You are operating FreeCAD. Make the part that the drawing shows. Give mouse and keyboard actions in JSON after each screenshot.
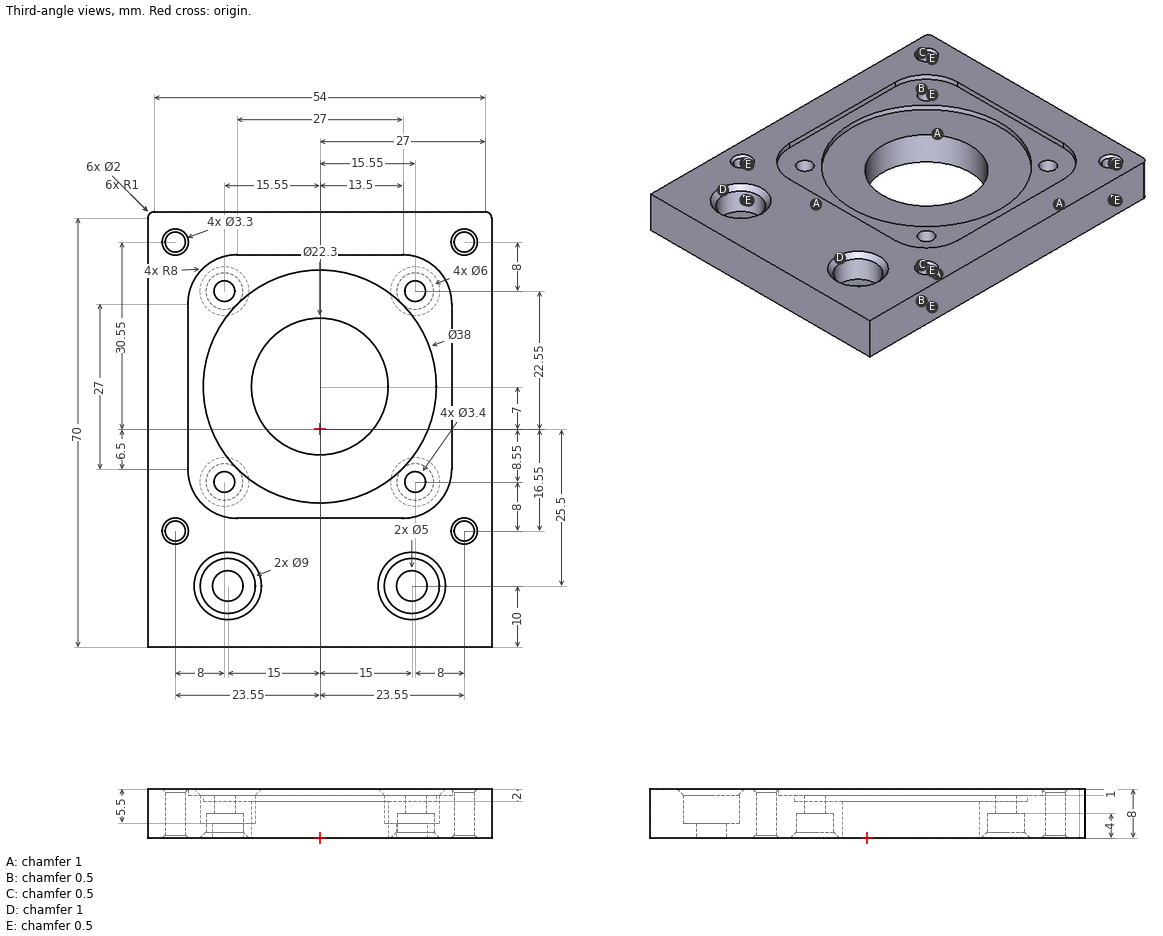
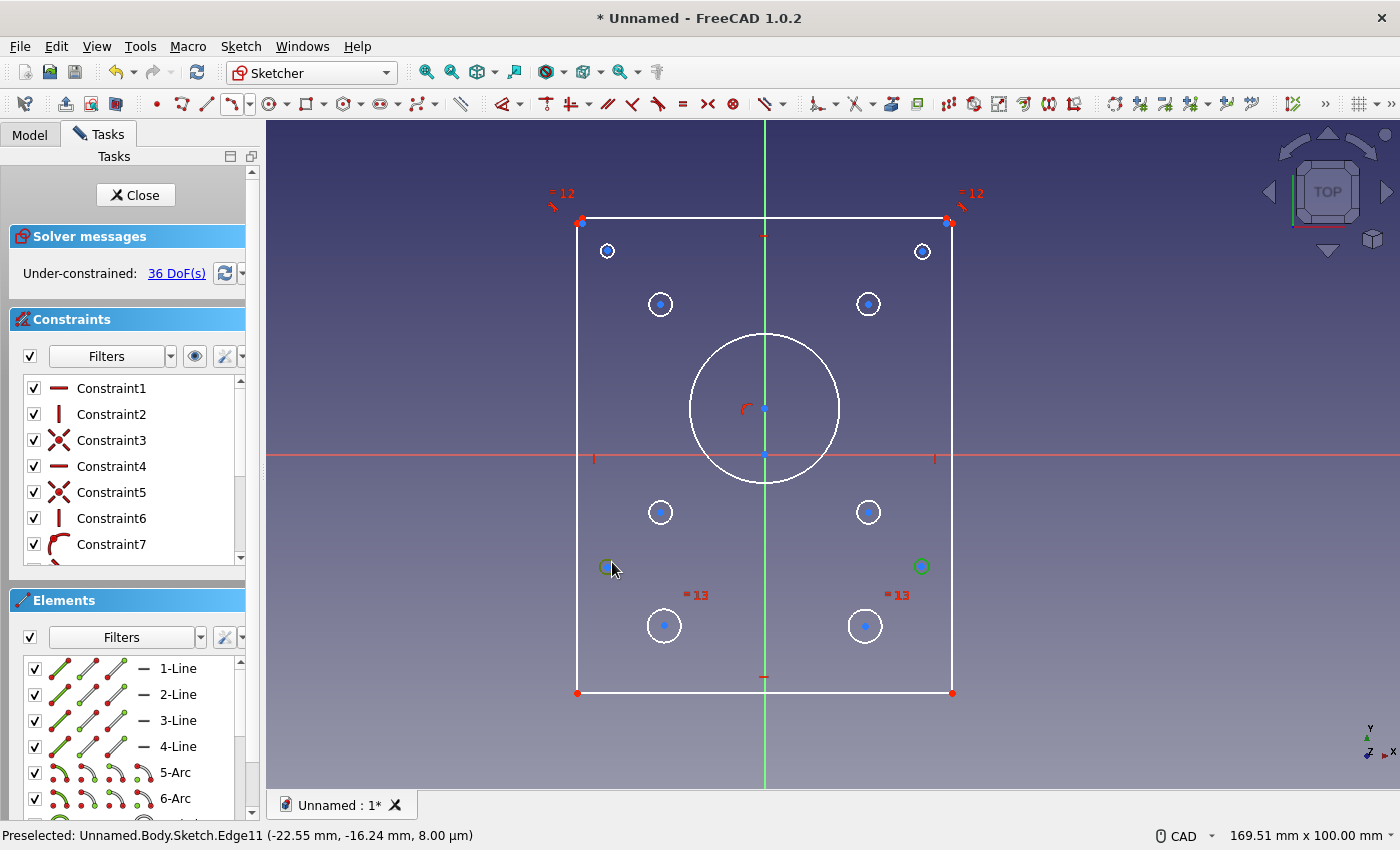
{"action": "scroll", "coordinate": [928, 247], "scroll_direction": "up", "scroll_amount": 4}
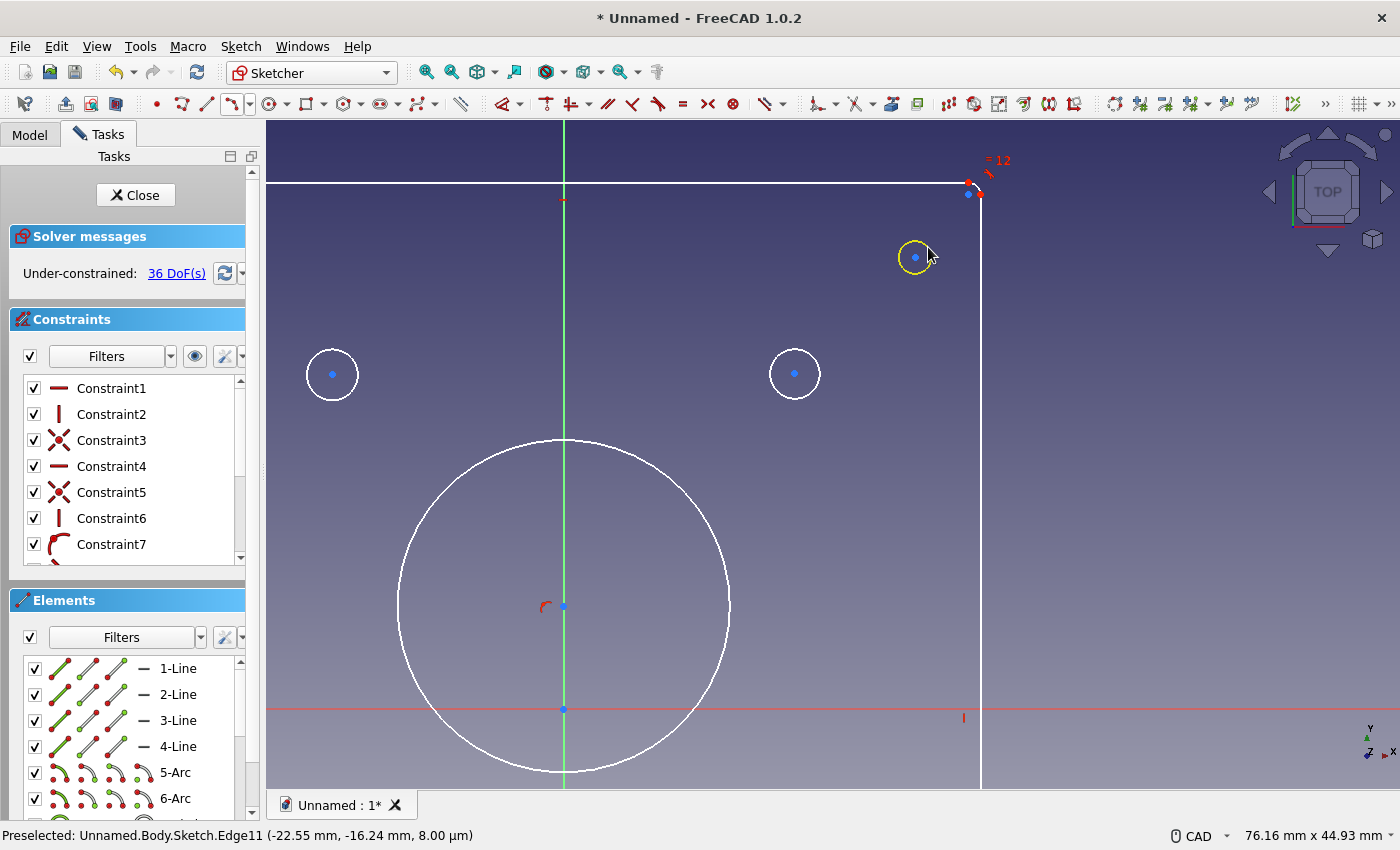
{"action": "left_click", "coordinate": [927, 246]}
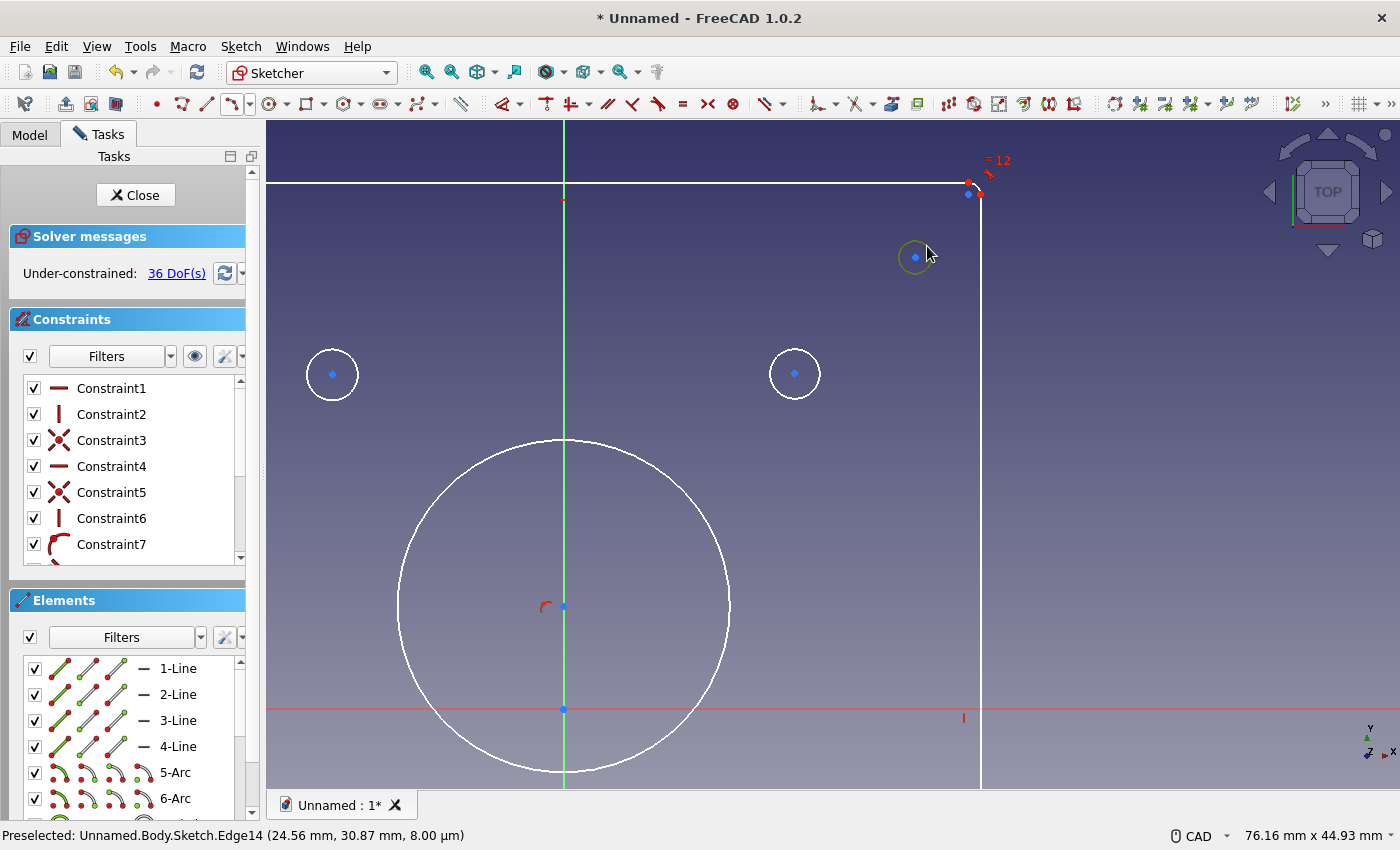
{"action": "scroll", "coordinate": [928, 247], "scroll_direction": "down", "scroll_amount": 4}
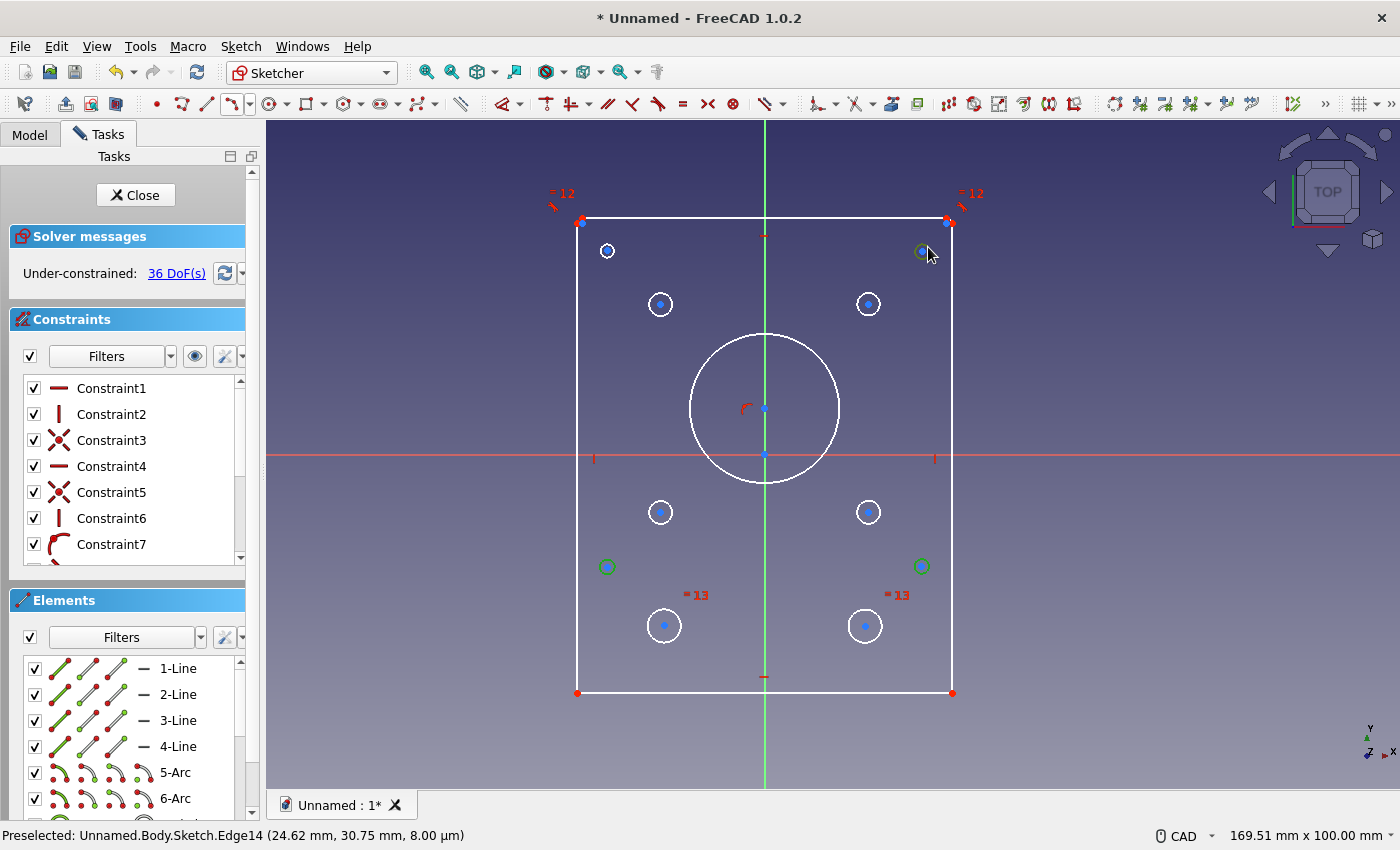
{"action": "scroll", "coordinate": [612, 246], "scroll_direction": "up", "scroll_amount": 4}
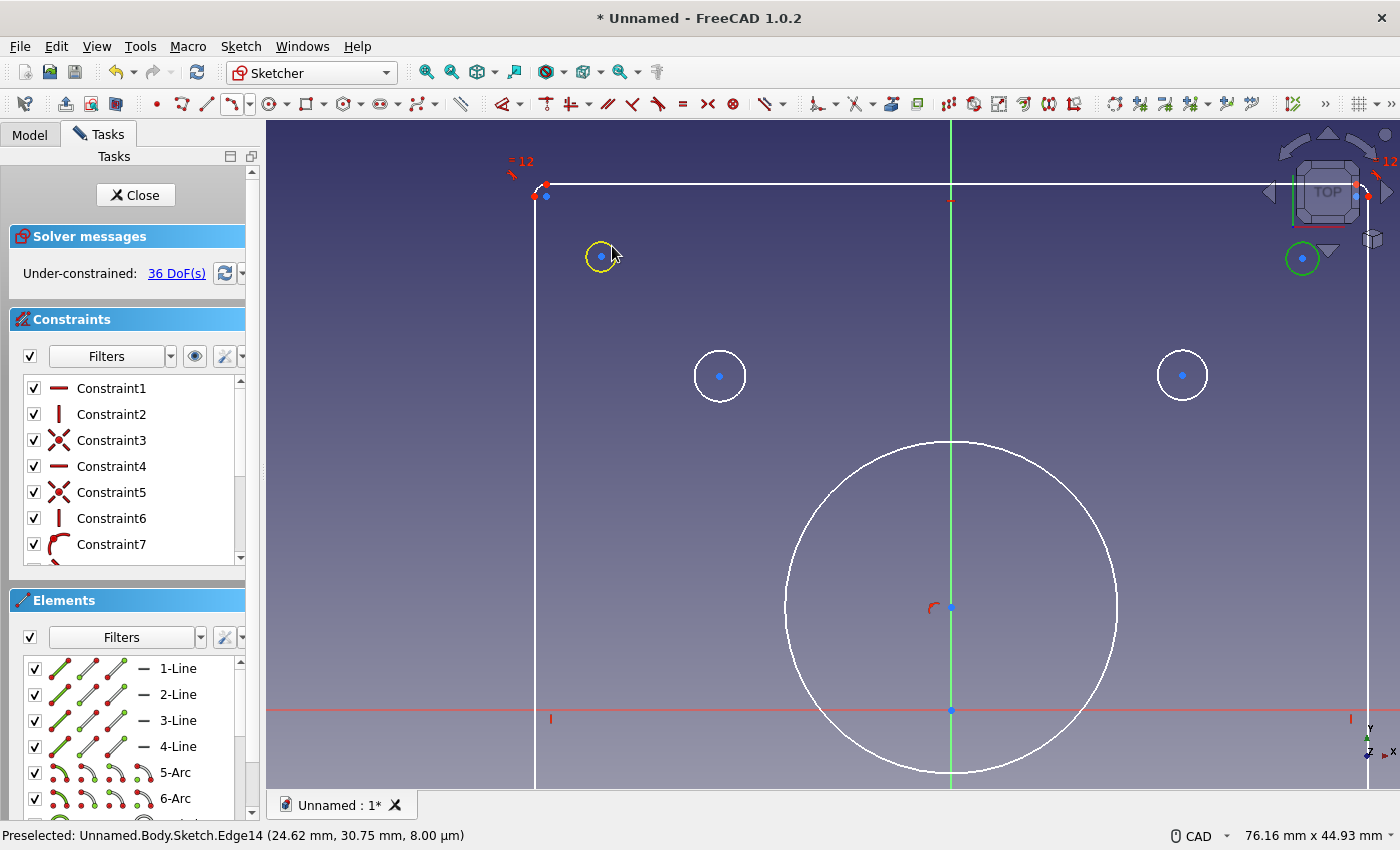
{"action": "left_click", "coordinate": [611, 246]}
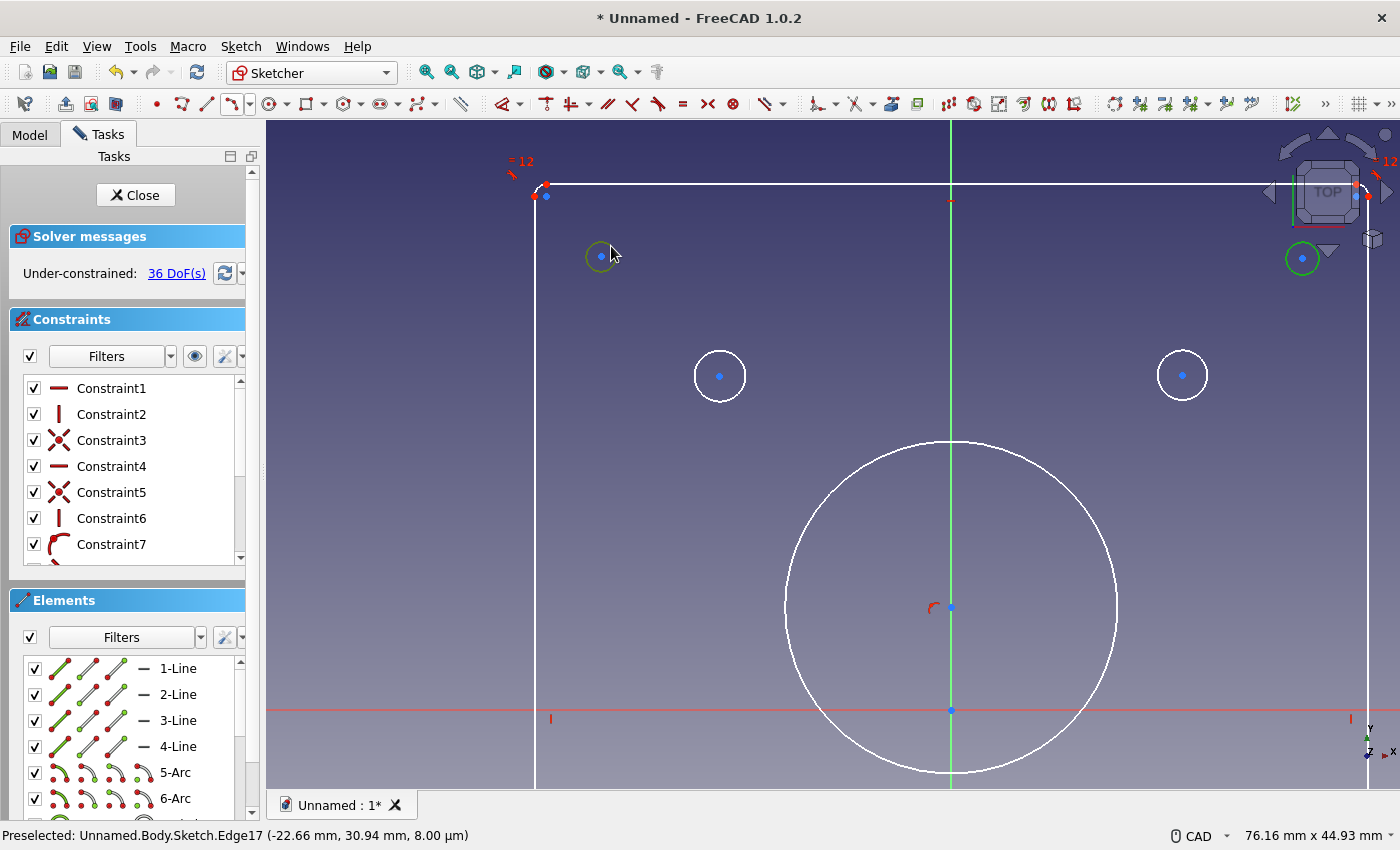
{"action": "key", "text": "e"}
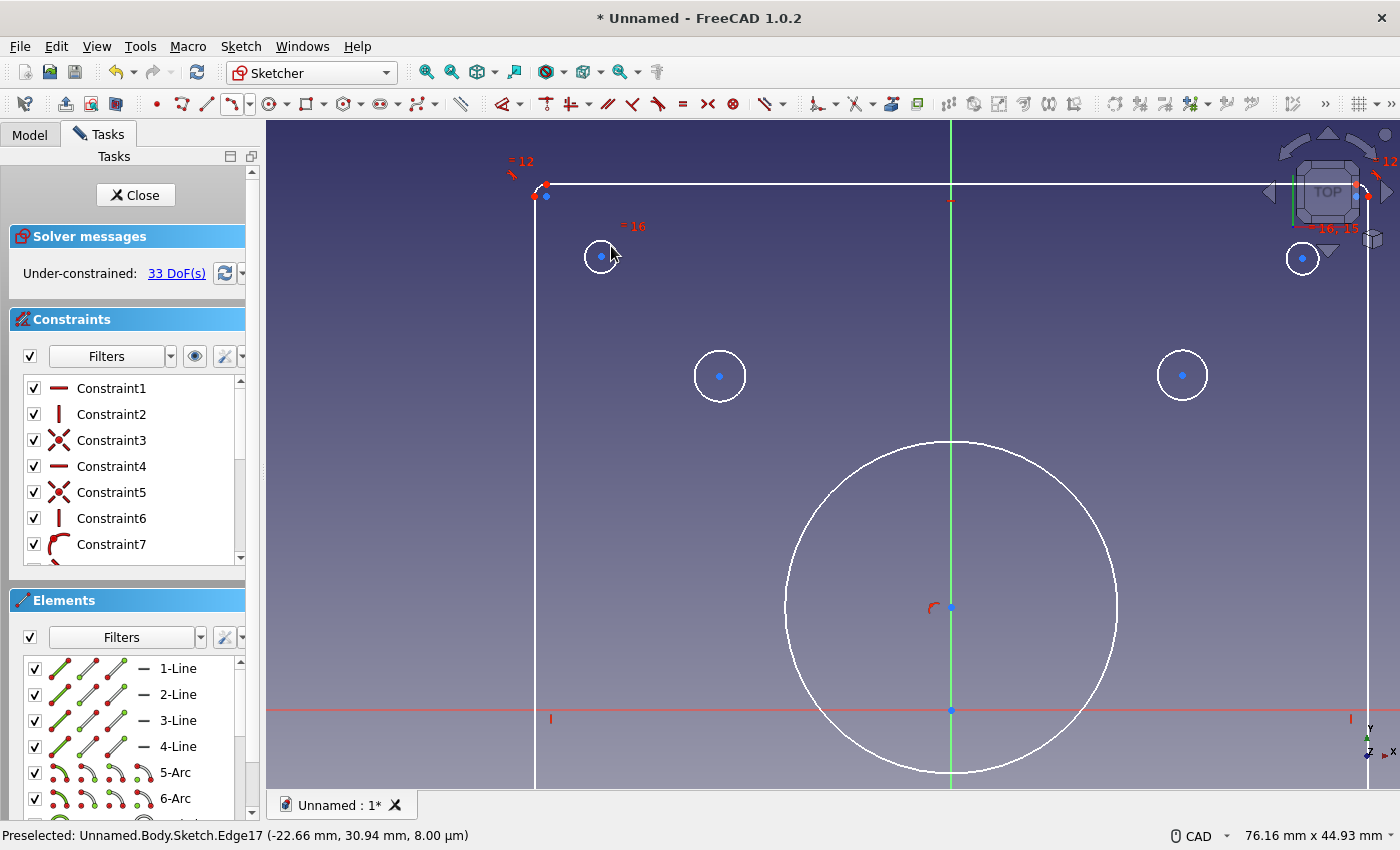
{"action": "scroll", "coordinate": [612, 246], "scroll_direction": "down", "scroll_amount": 4}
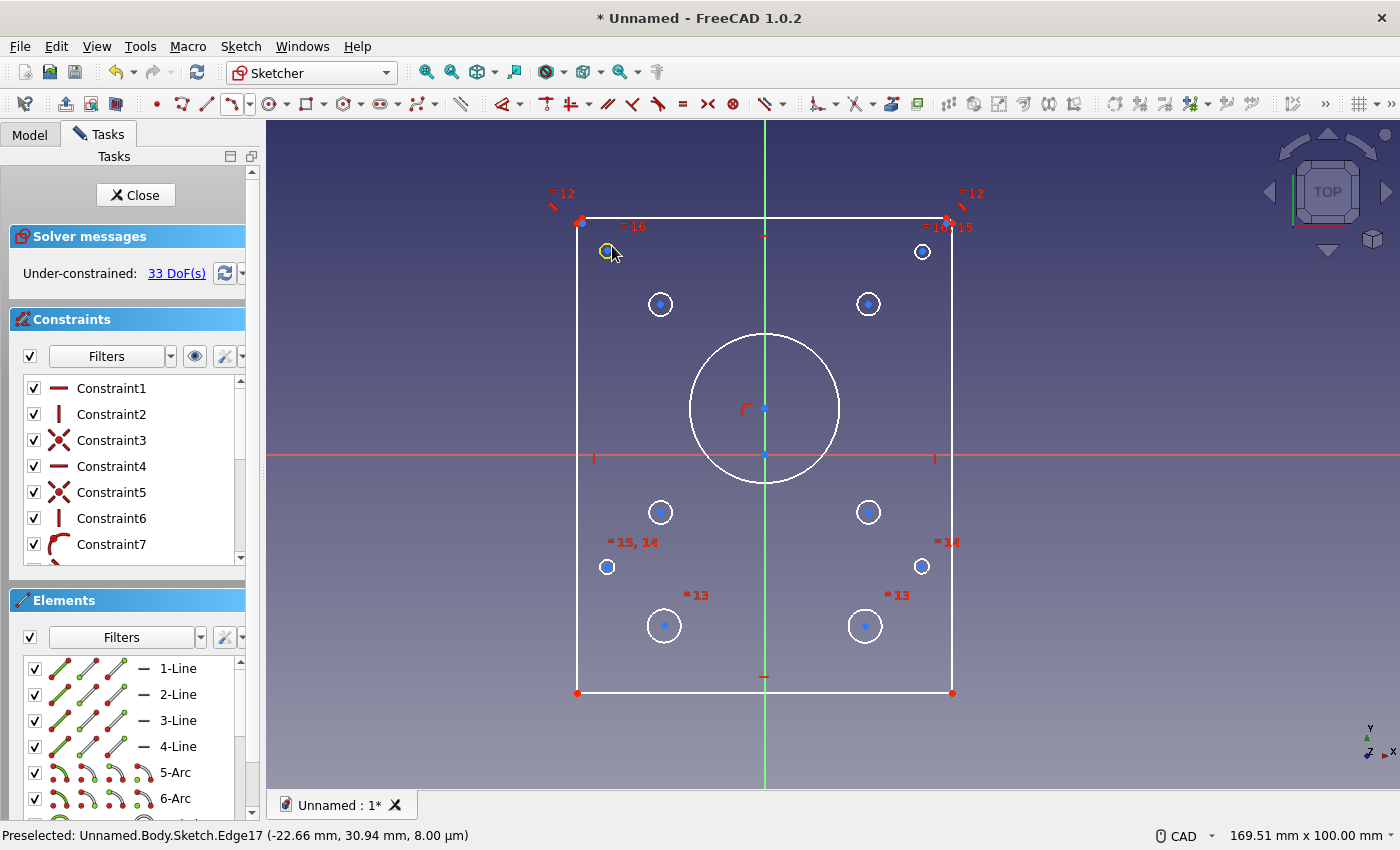
{"action": "left_click", "coordinate": [877, 504]}